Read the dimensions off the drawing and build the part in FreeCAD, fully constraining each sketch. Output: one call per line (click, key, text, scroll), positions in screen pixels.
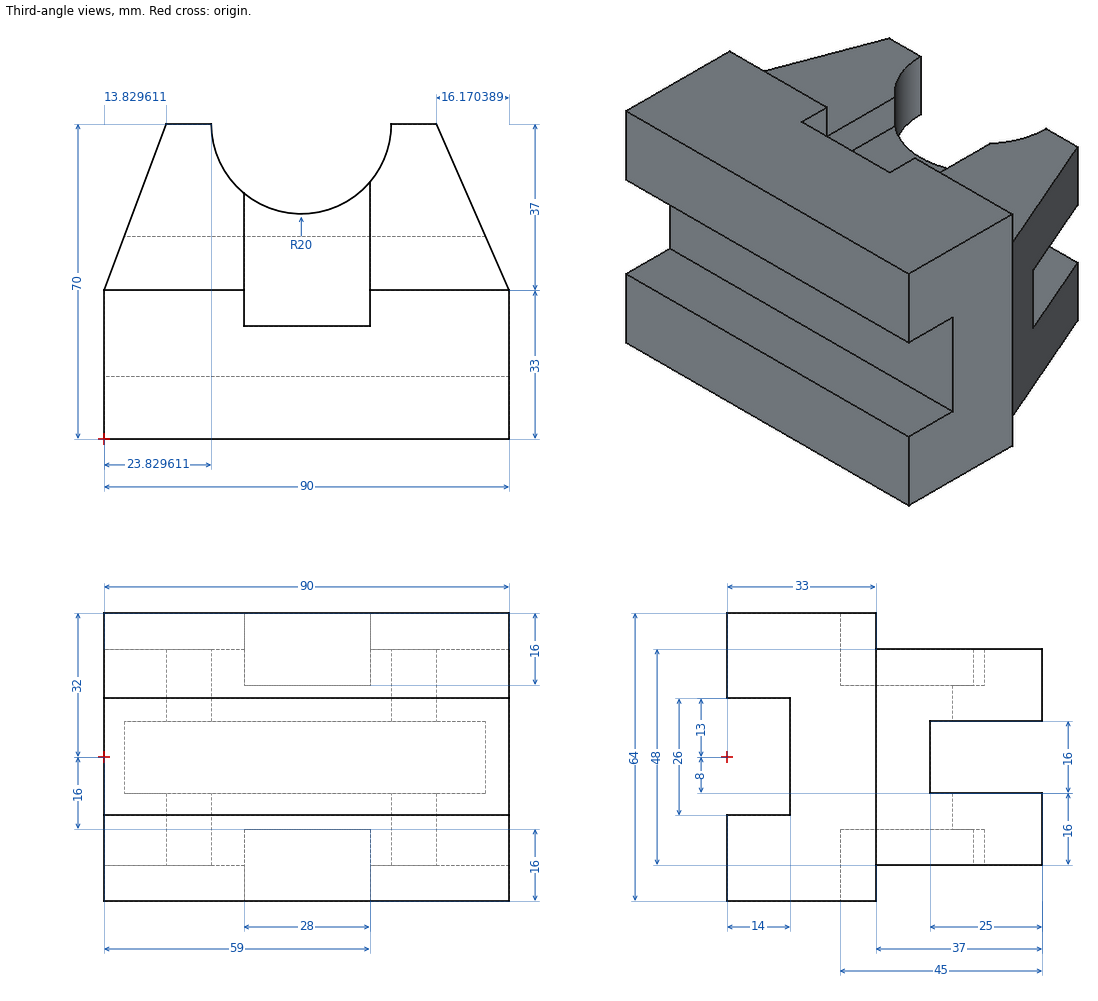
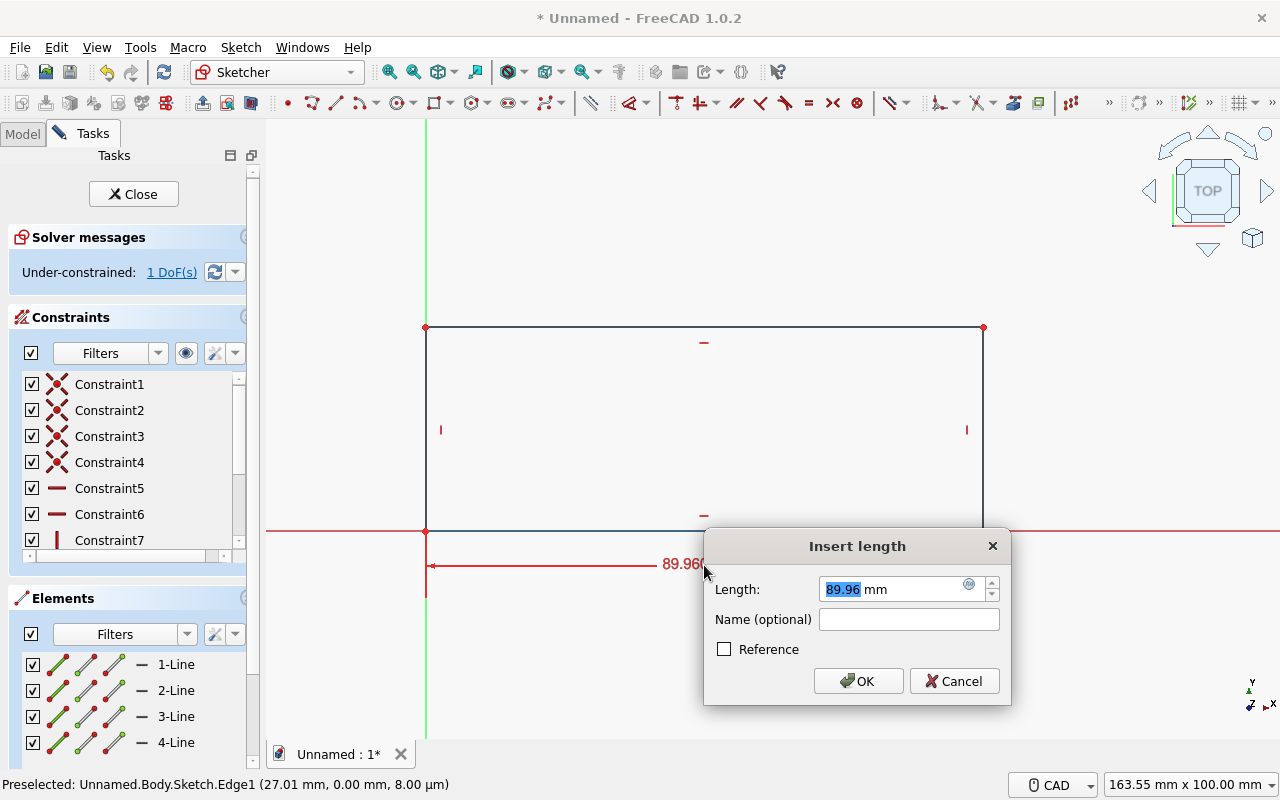
text(90)
key(Return)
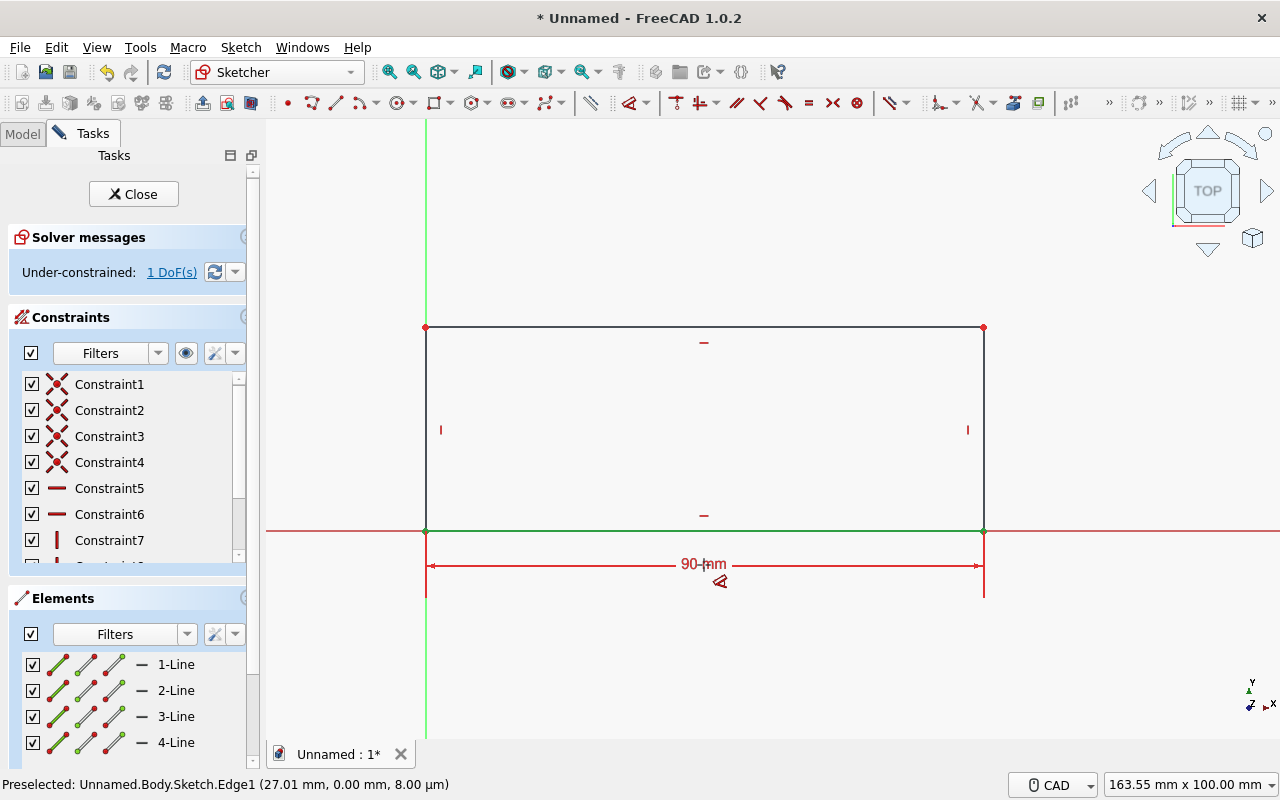
click(984, 470)
click(1018, 429)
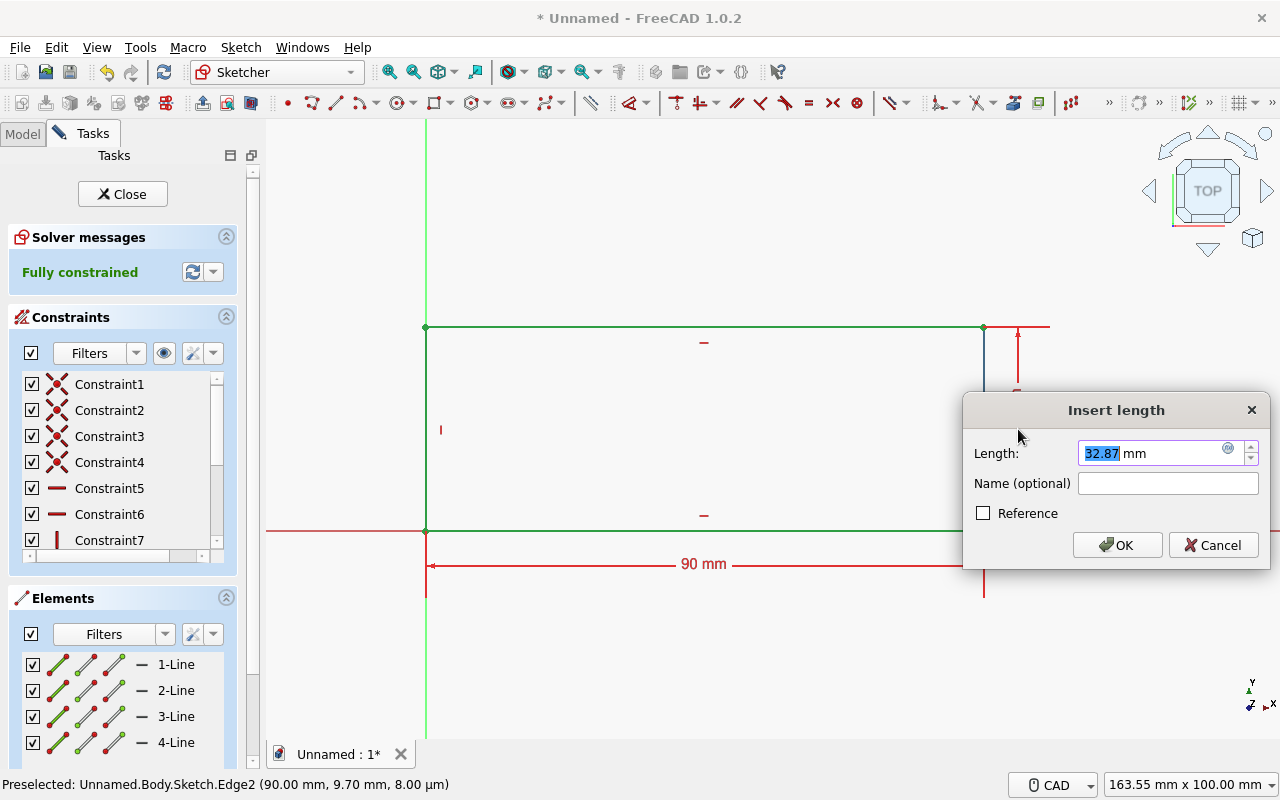
text(33)
key(Return)
key(Escape)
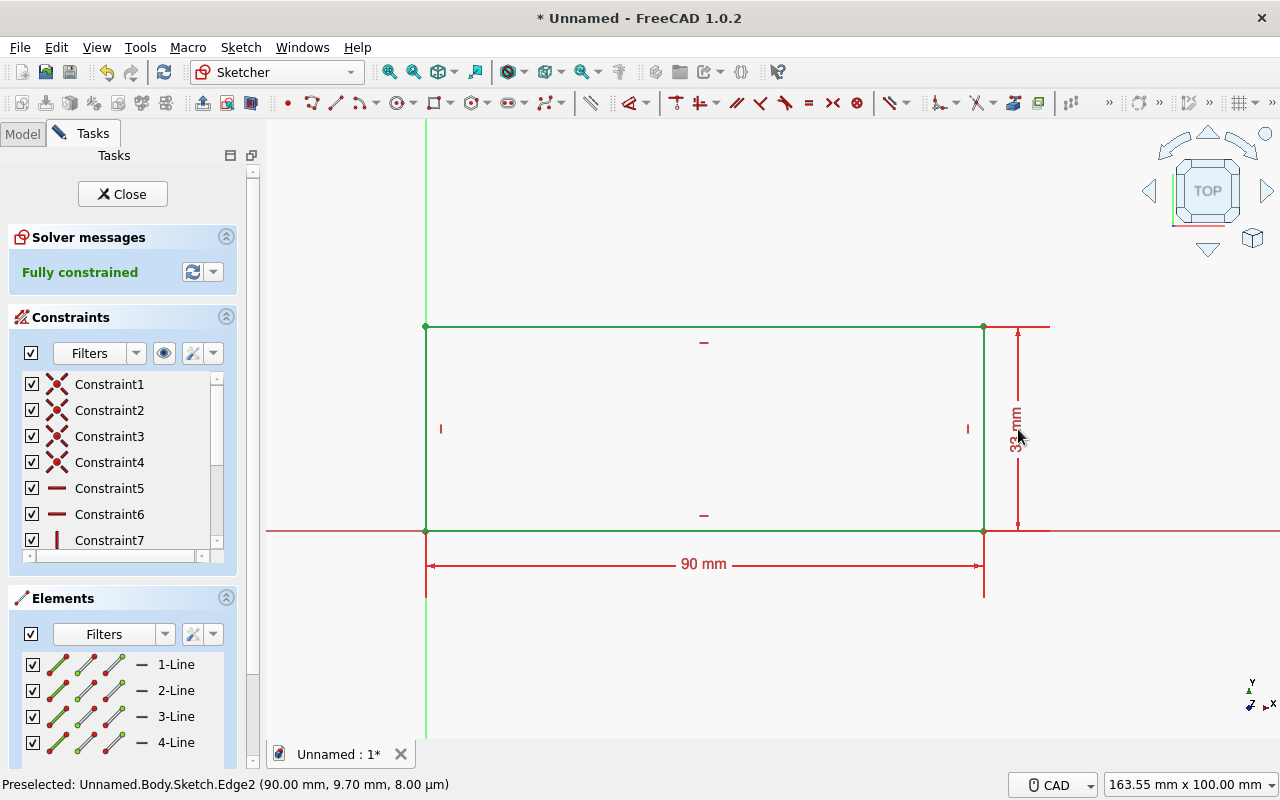
click(123, 194)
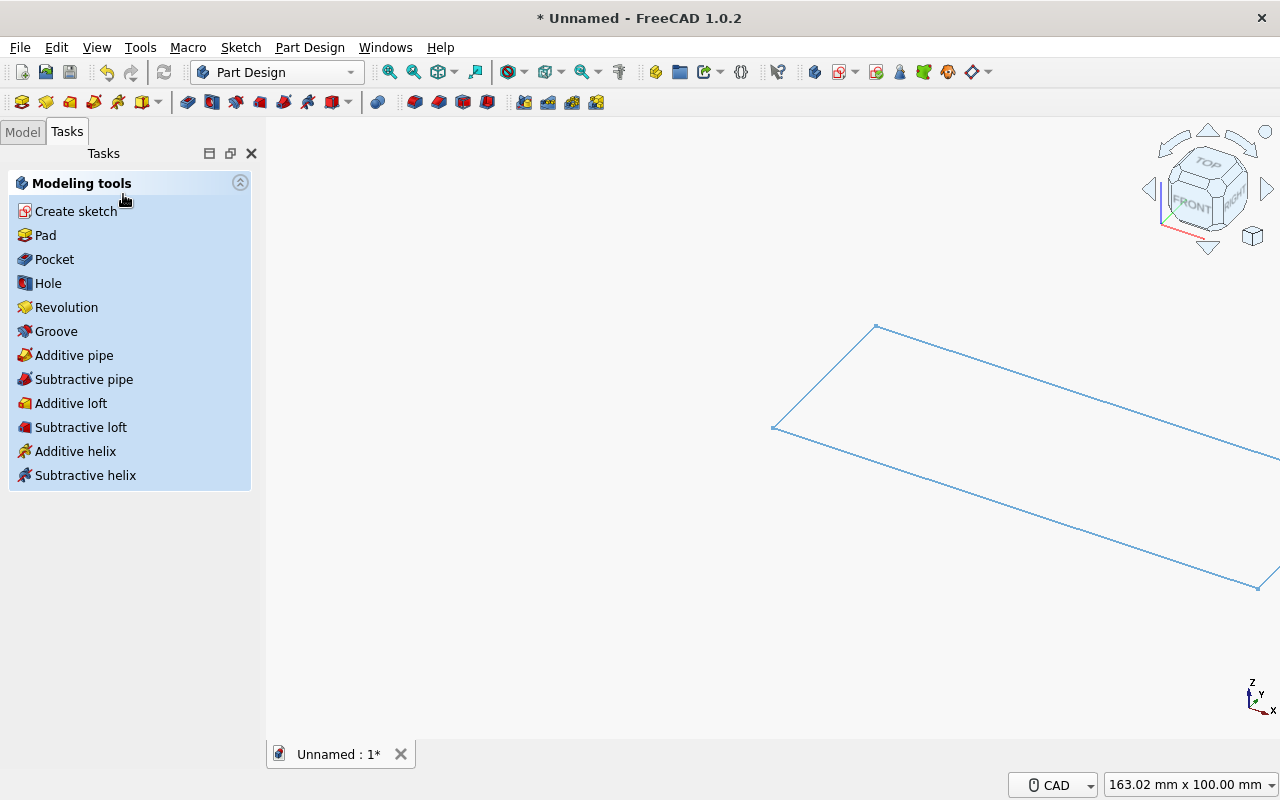
click(22, 102)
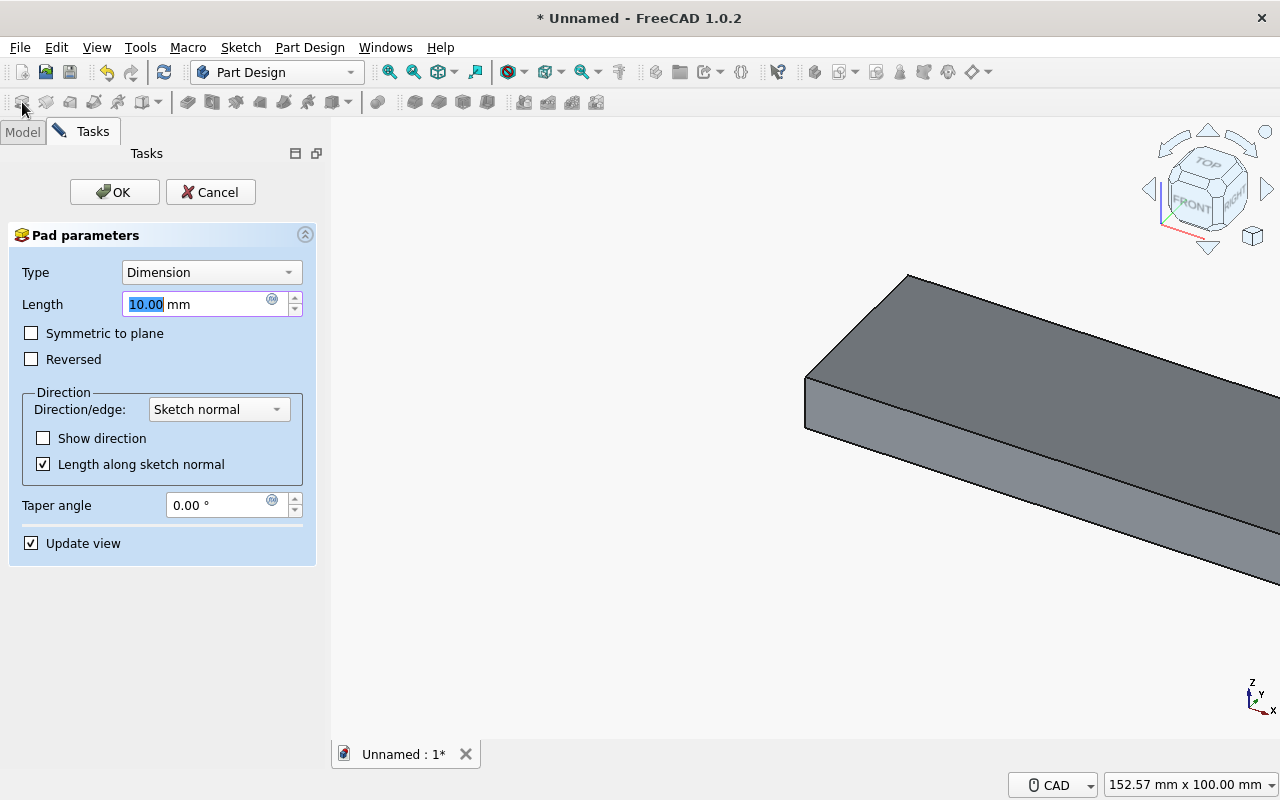
text(64)
key(Tab)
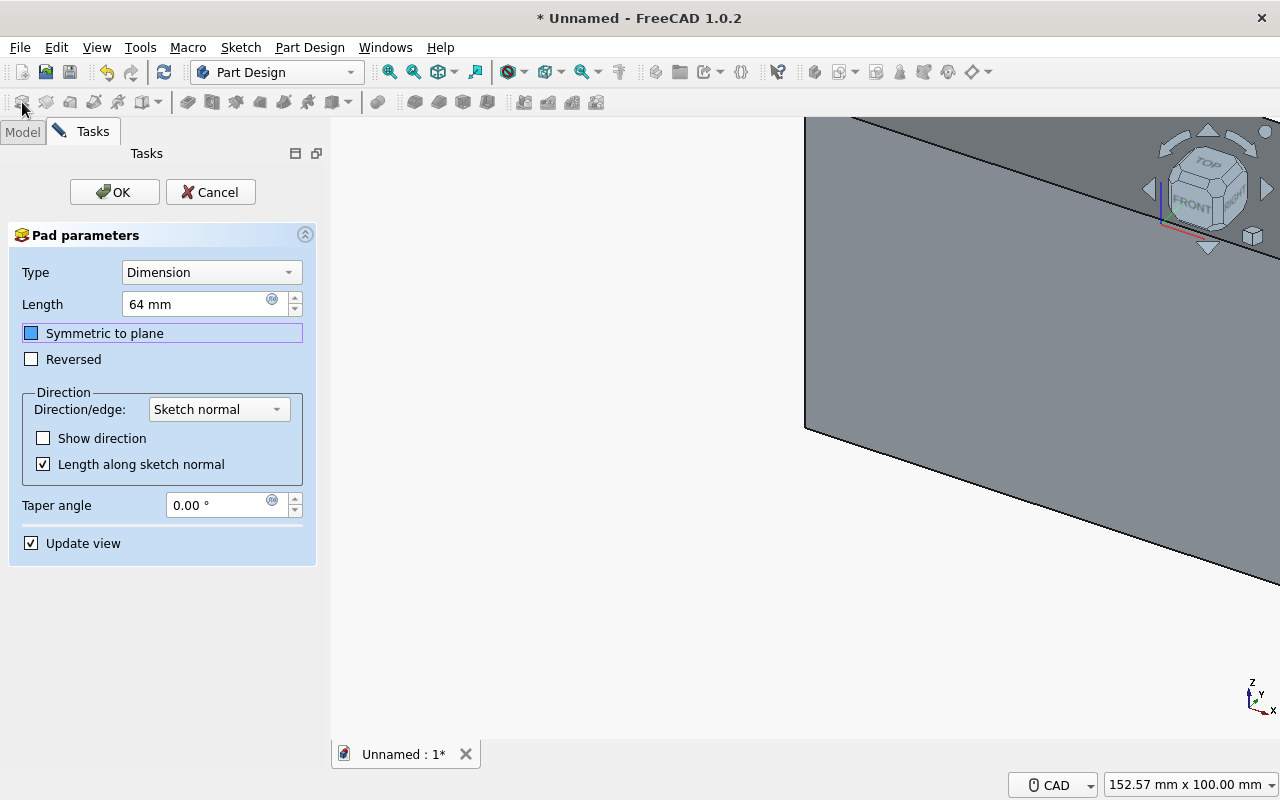
click(30, 333)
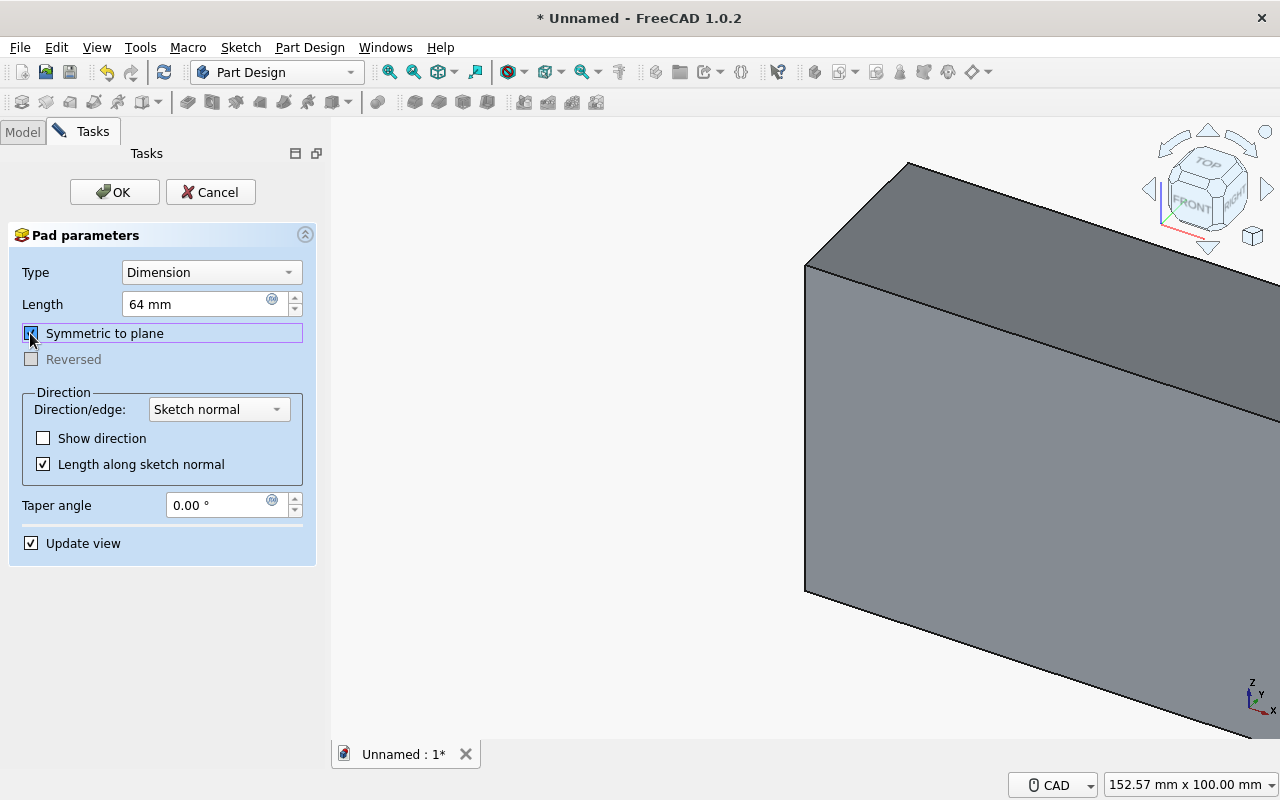
click(115, 192)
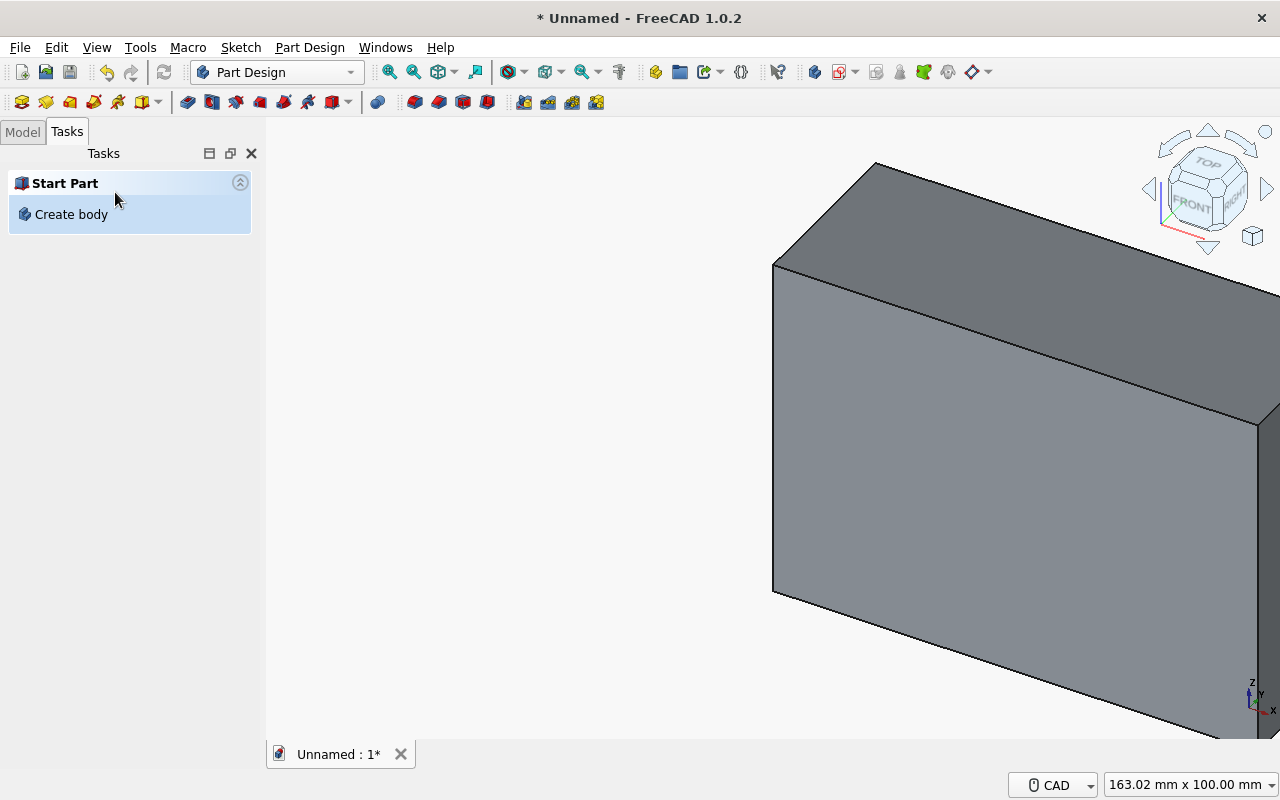
key(v)
key(f)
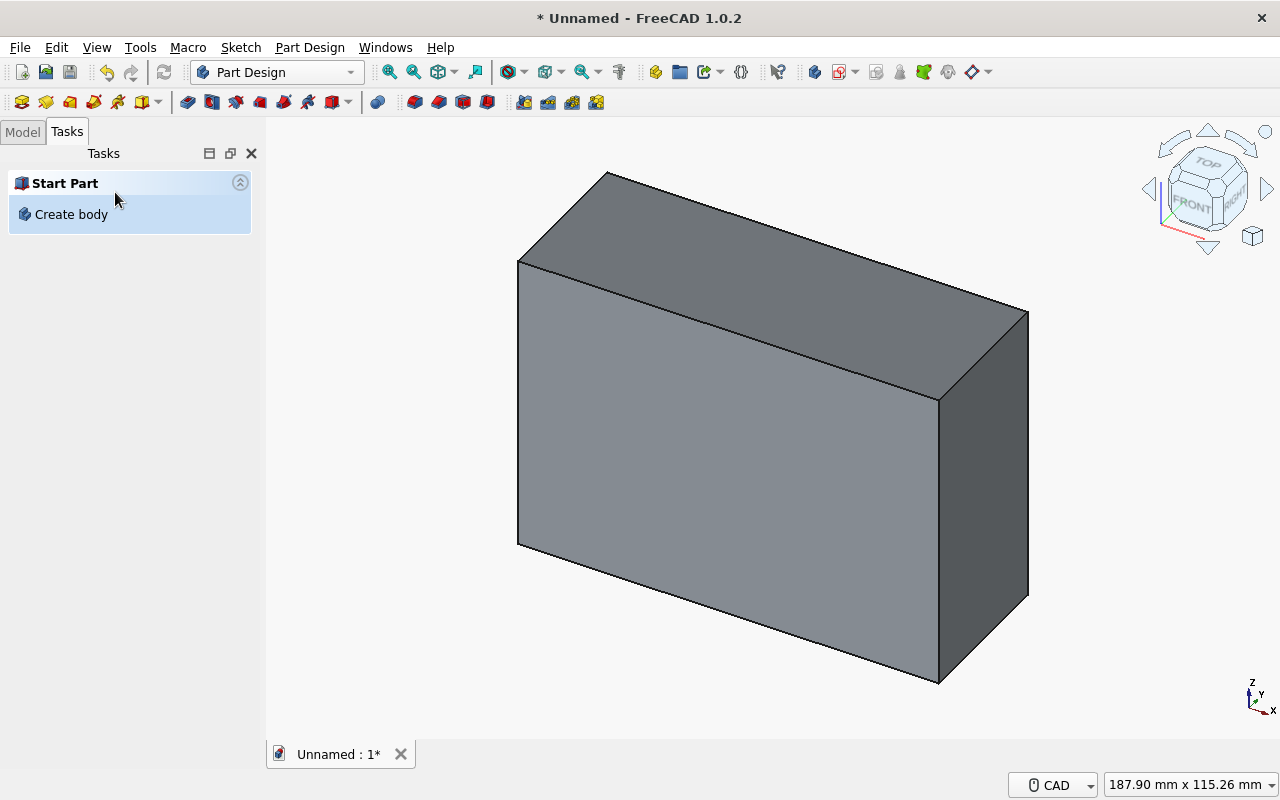
click(983, 456)